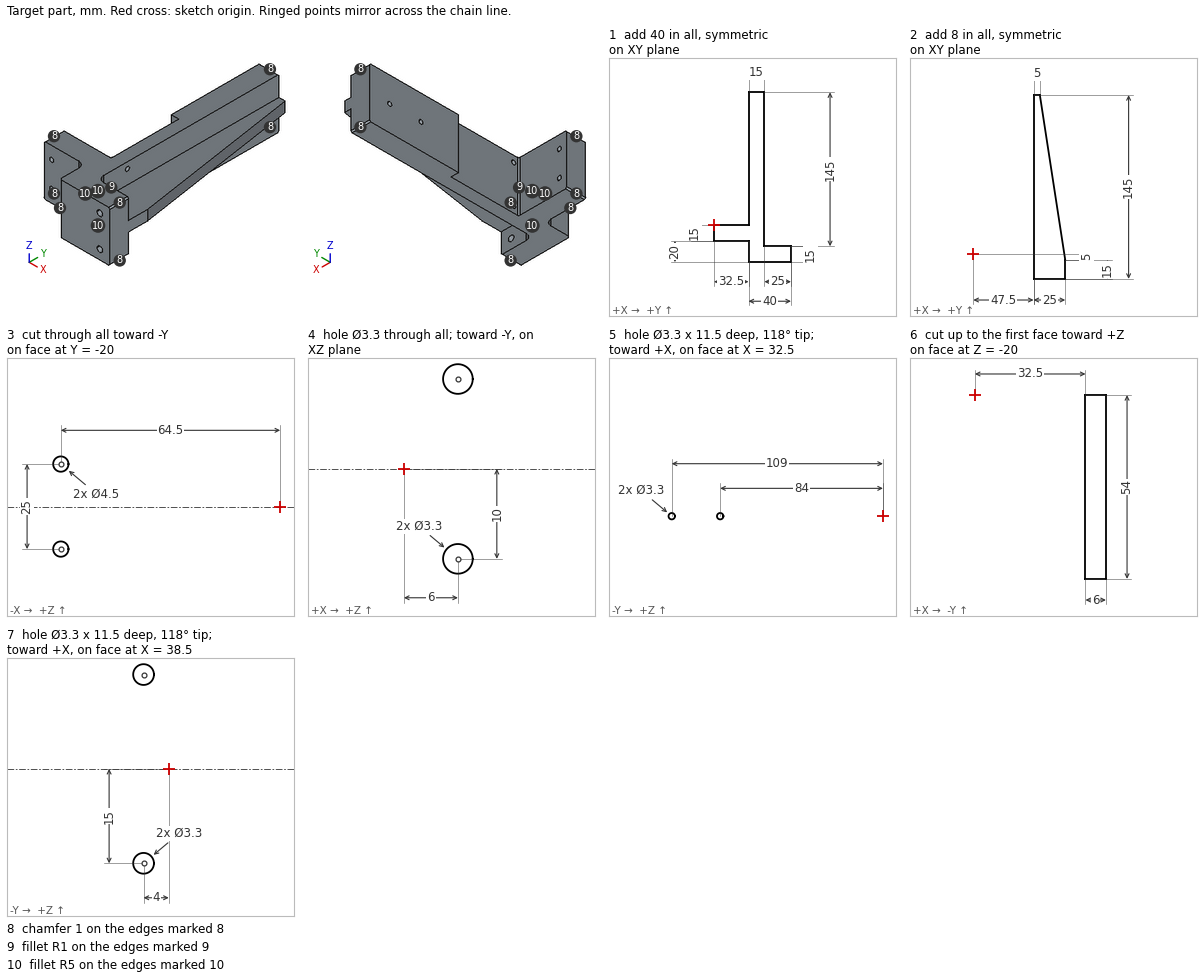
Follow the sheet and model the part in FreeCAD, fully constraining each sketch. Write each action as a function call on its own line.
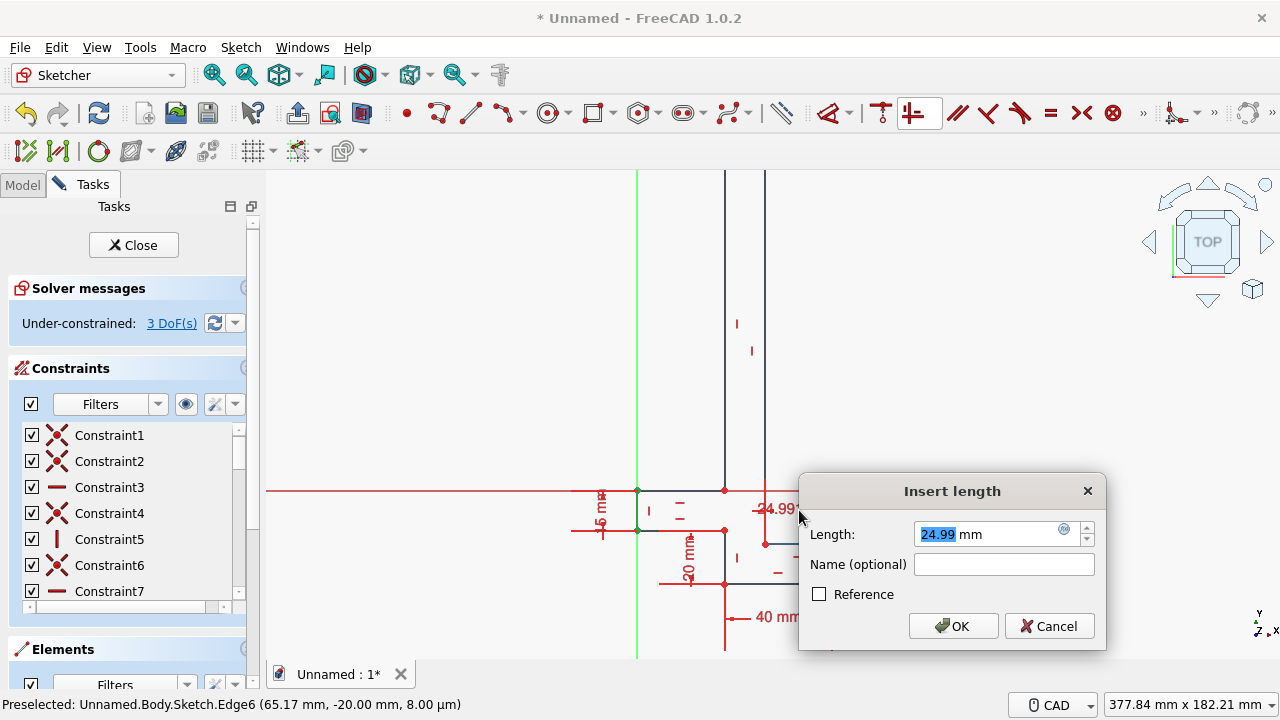
text(25)
key(Return)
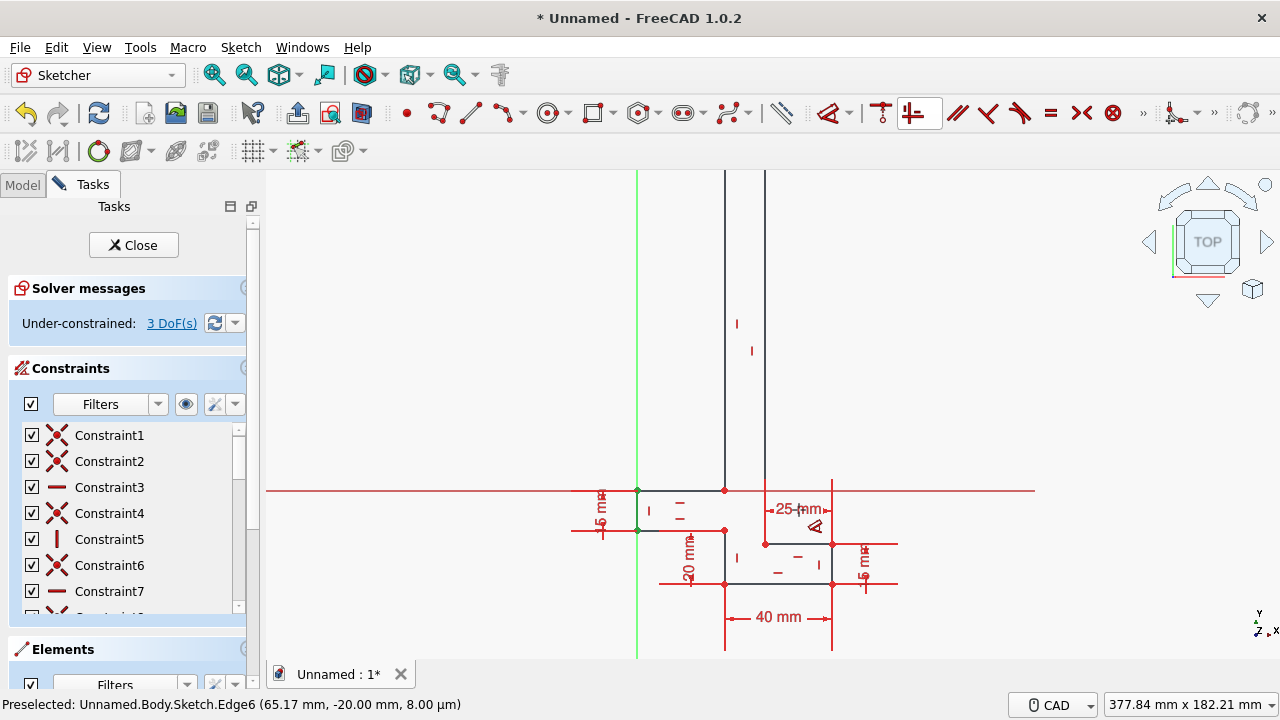
scroll(644, 505, down, 2)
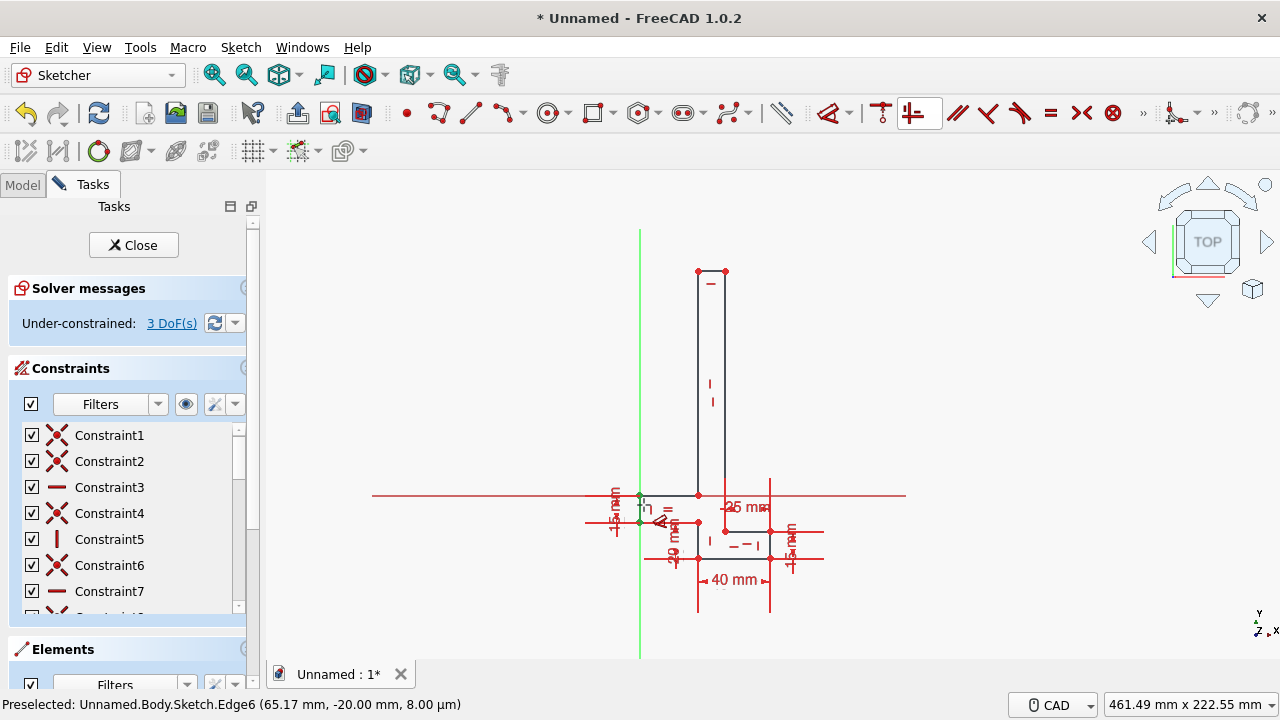
scroll(717, 271, up, 3)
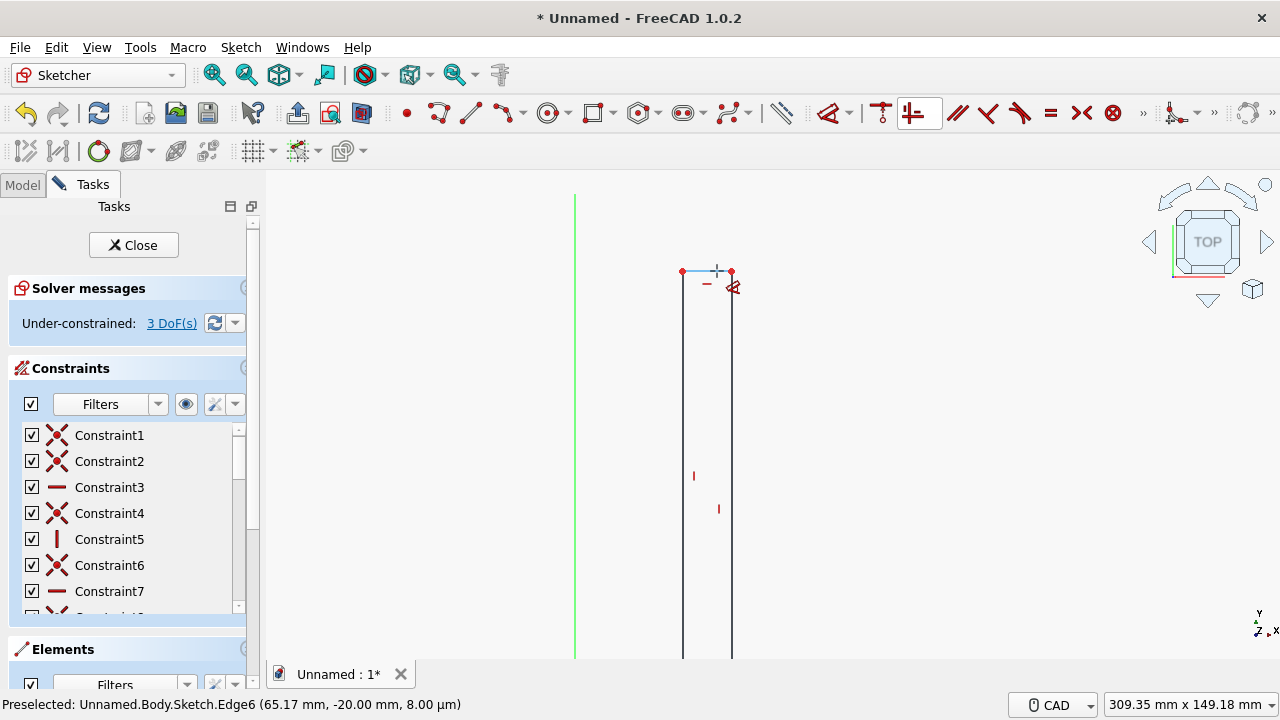
click(717, 271)
click(707, 237)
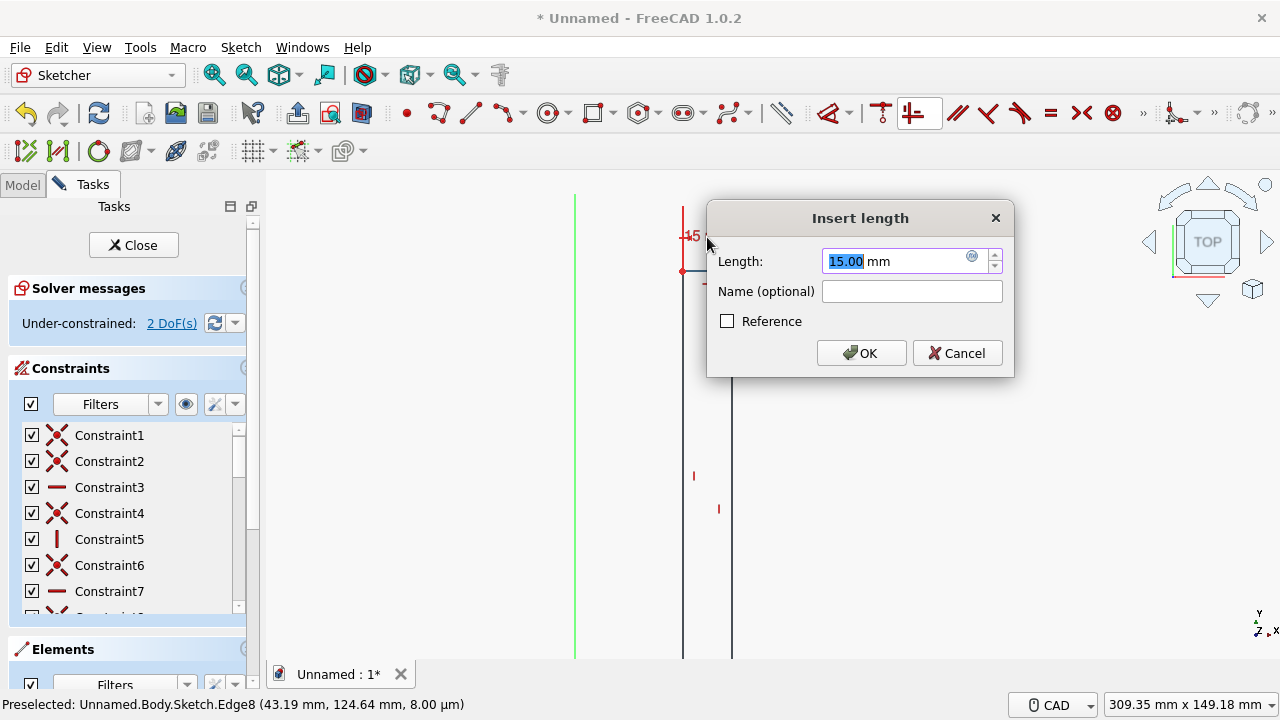
text(15)
key(Return)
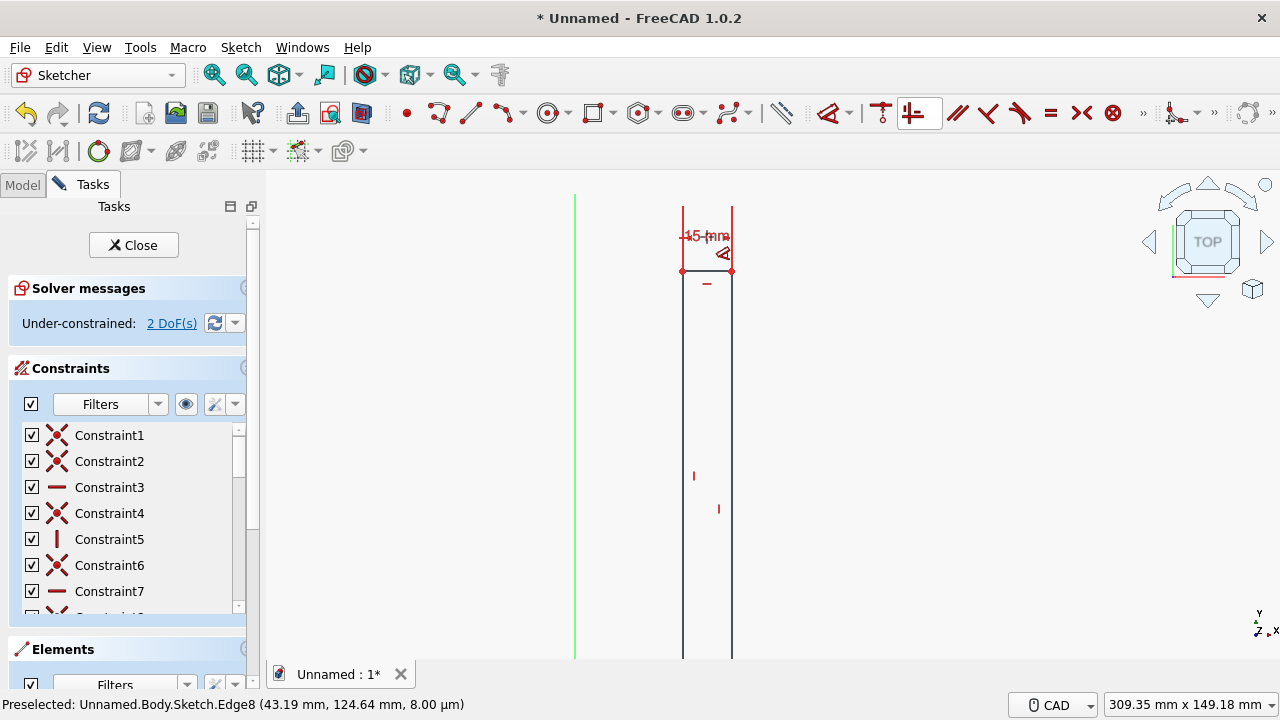
click(732, 603)
click(766, 451)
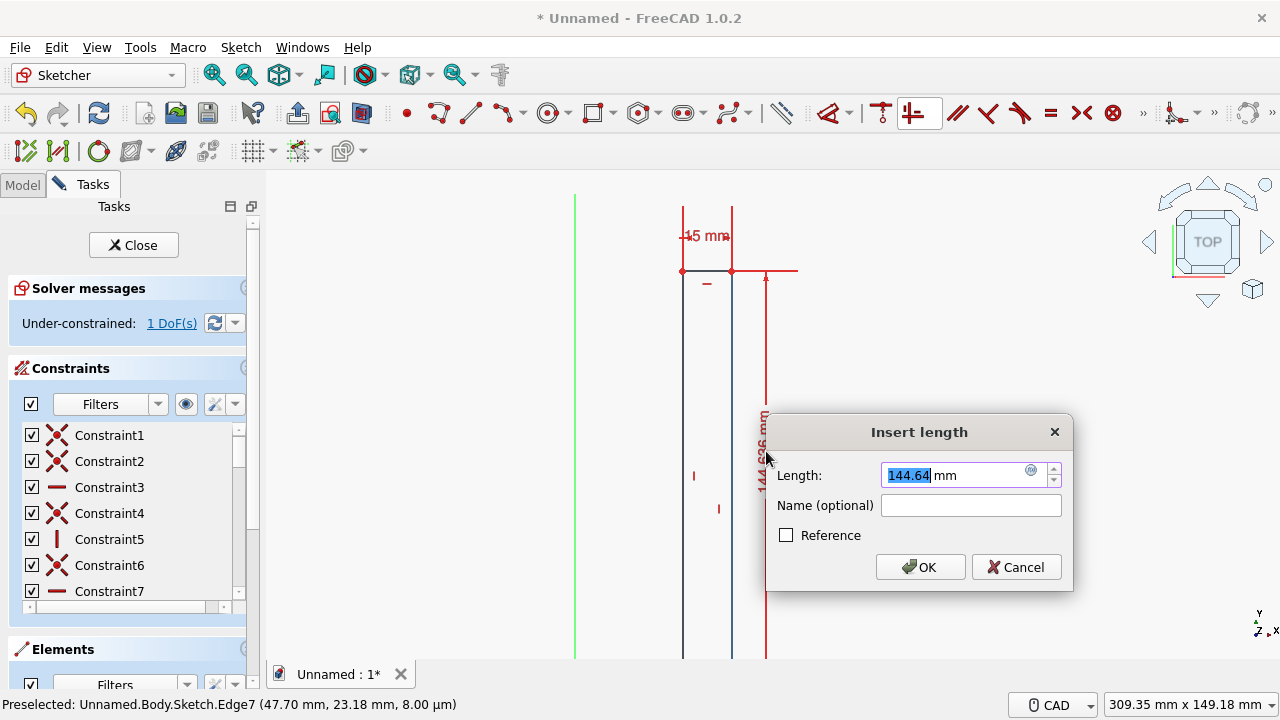
text(145)
key(Return)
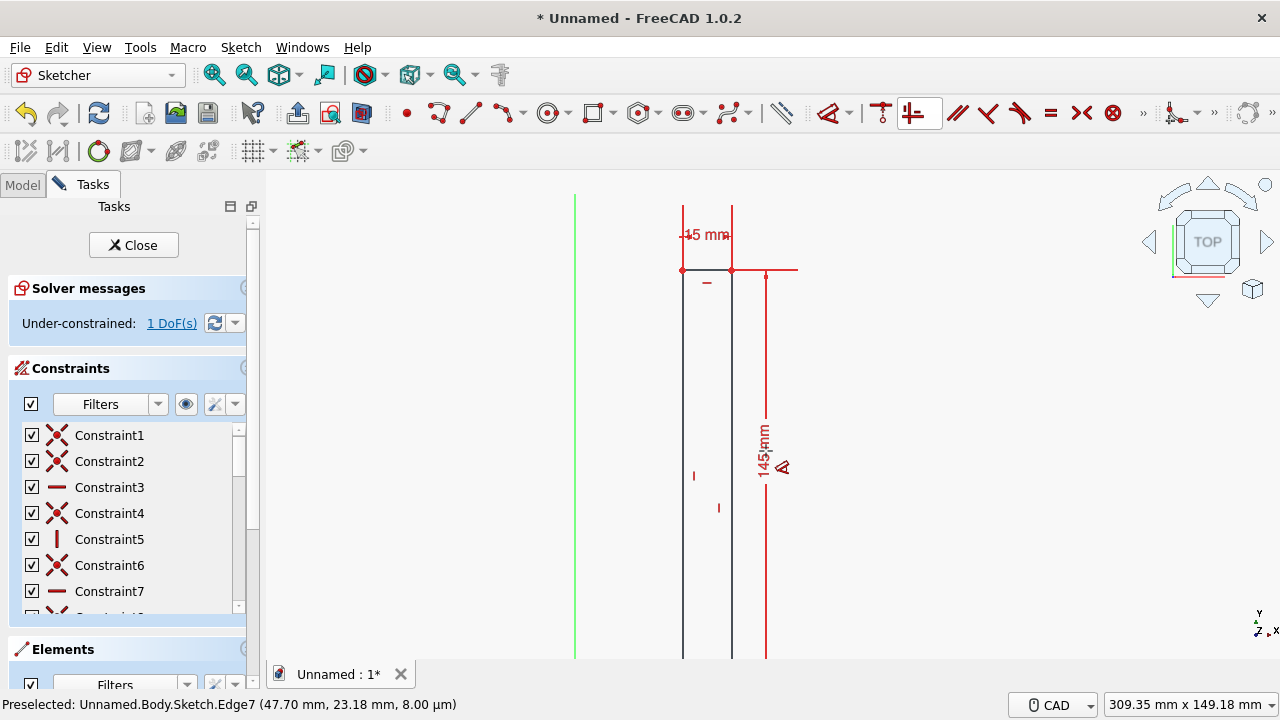
scroll(717, 271, down, 3)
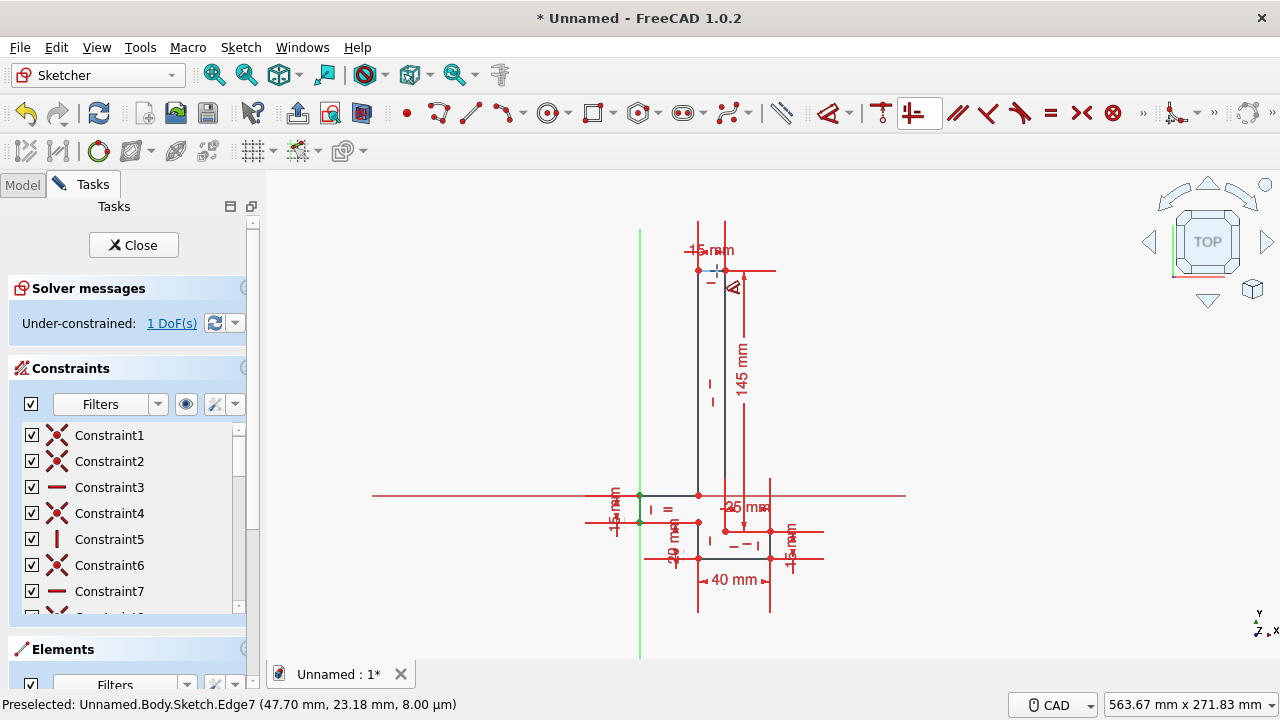
click(657, 523)
click(655, 581)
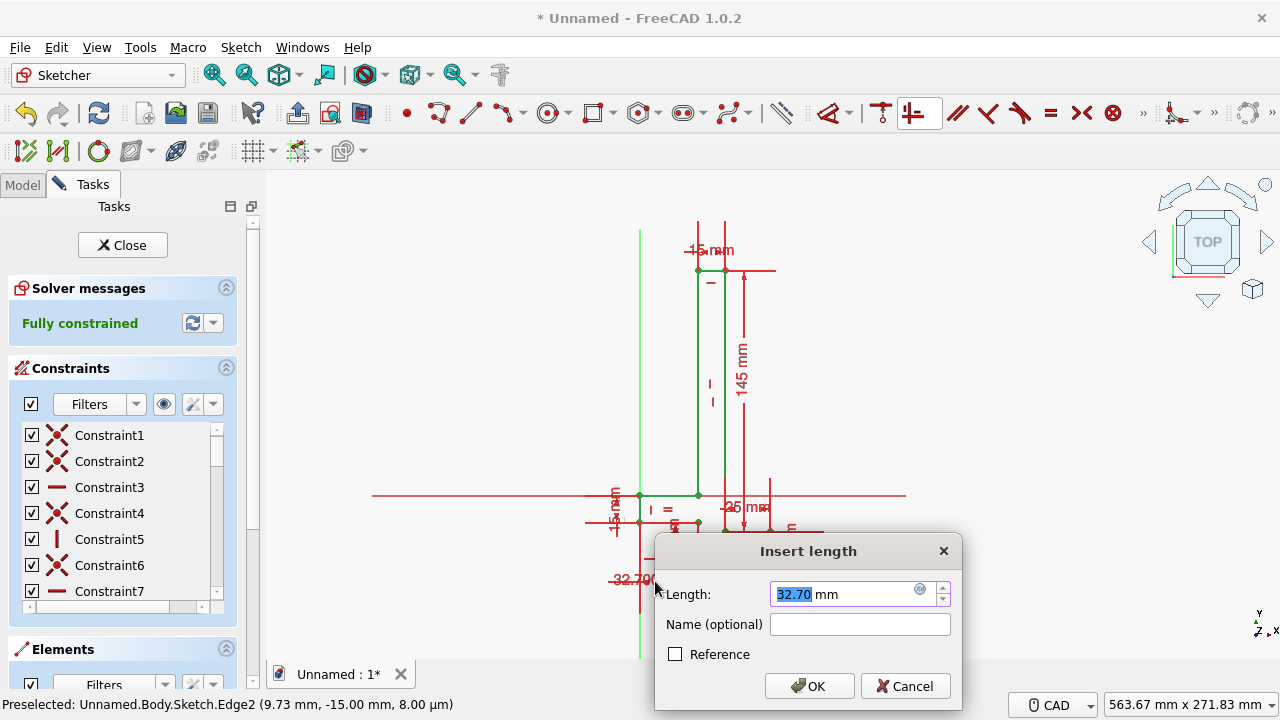
text(32.5)
key(Return)
key(Escape)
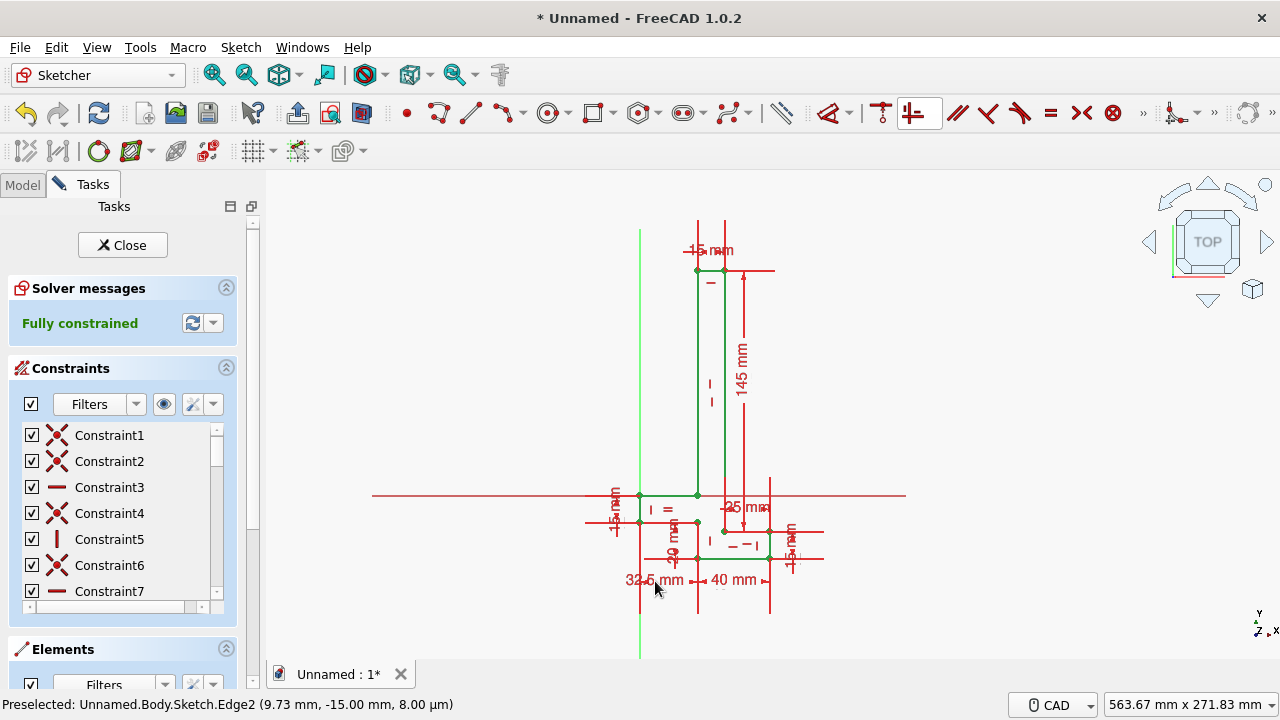
click(123, 245)